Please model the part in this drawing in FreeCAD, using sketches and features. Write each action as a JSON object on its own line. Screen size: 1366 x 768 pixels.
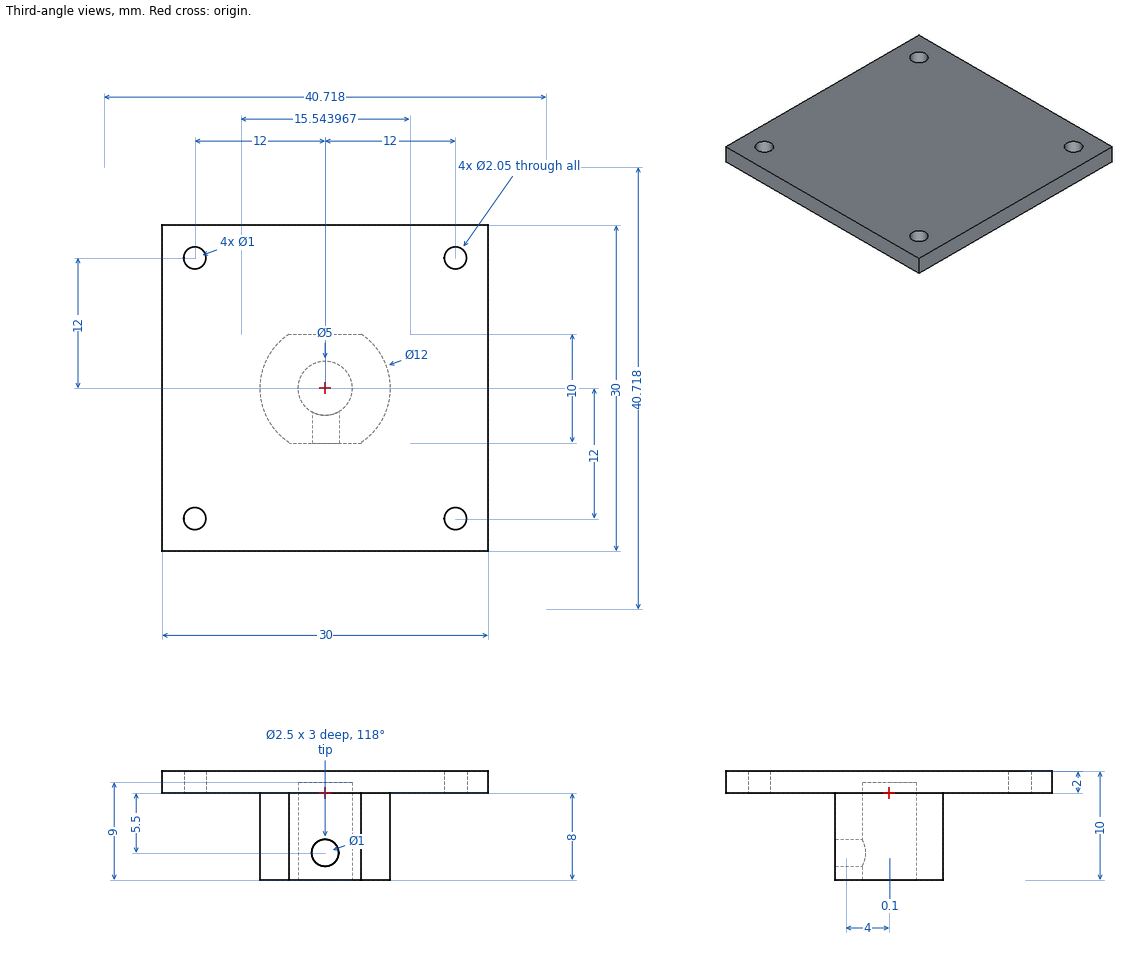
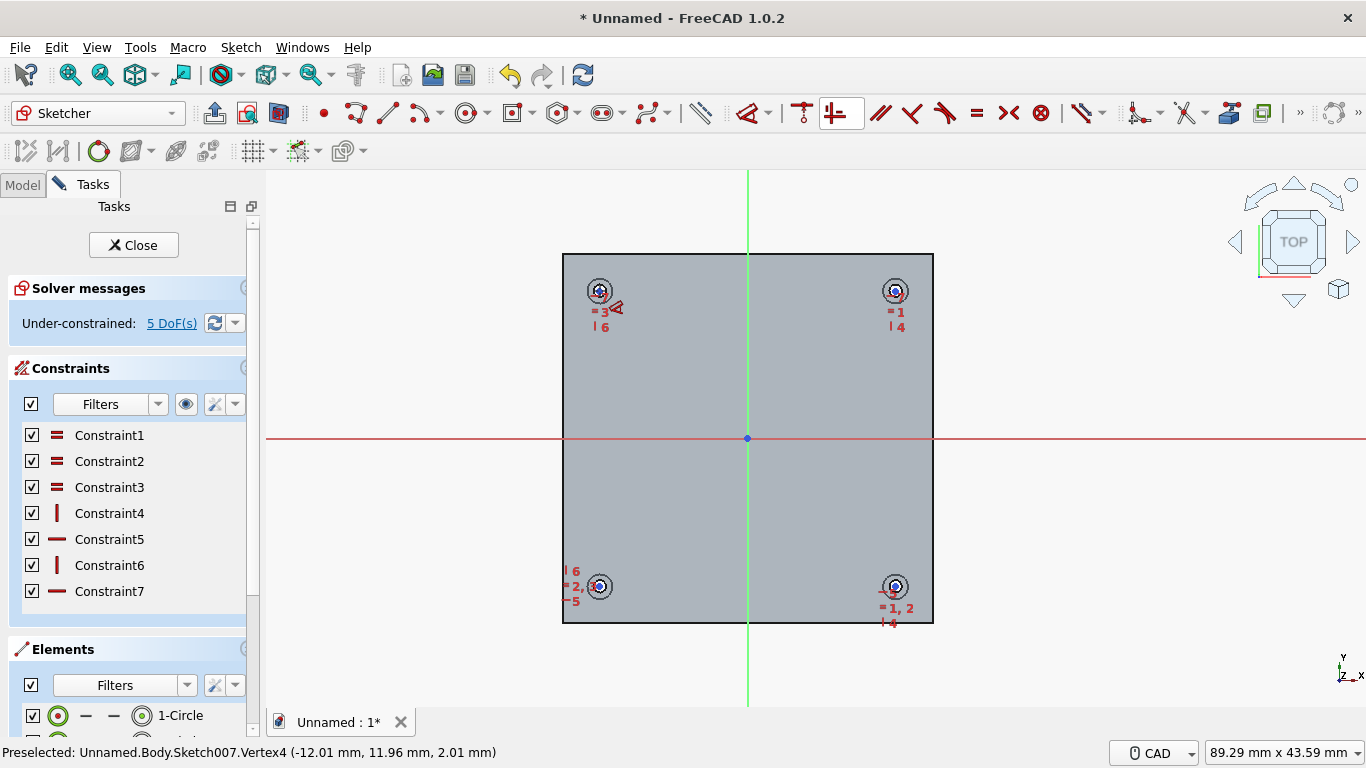
{"action": "scroll", "coordinate": [904, 282], "scroll_direction": "up", "scroll_amount": 3}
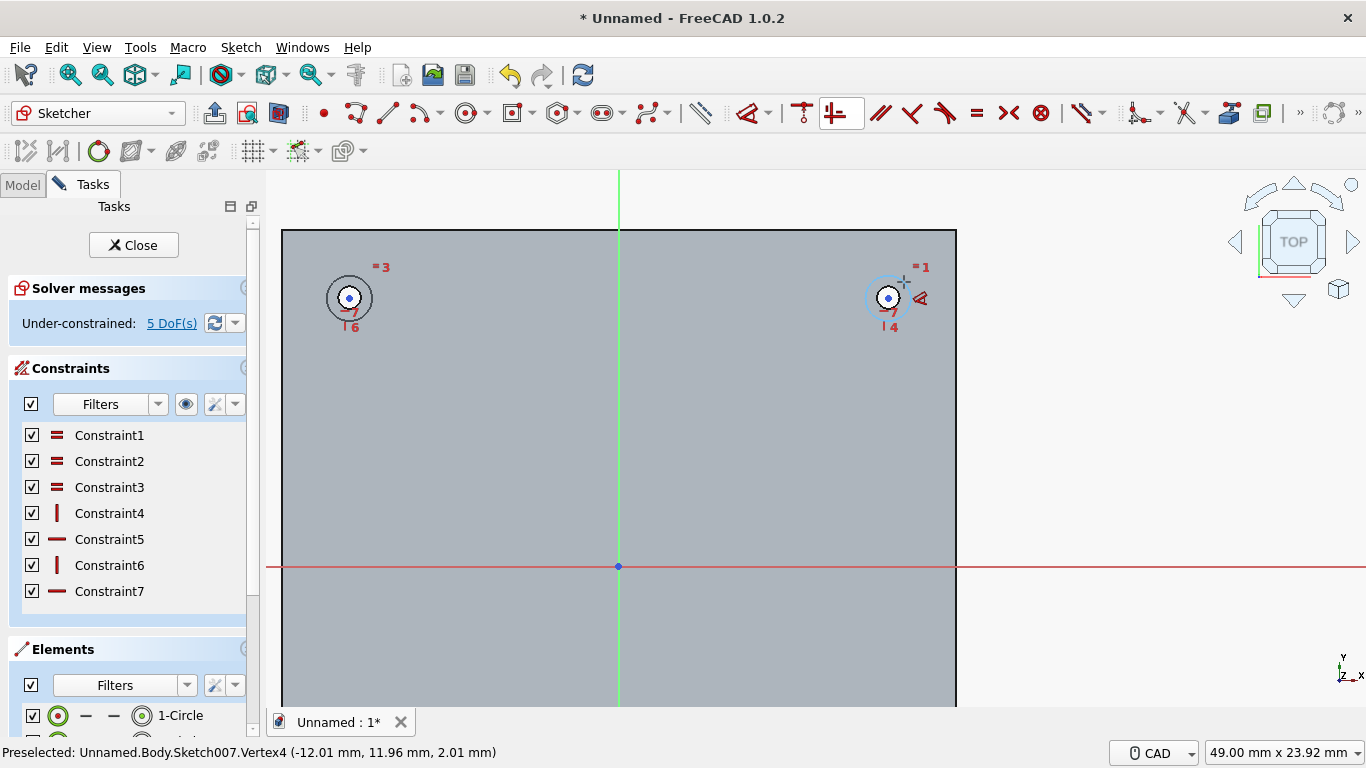
{"action": "left_click", "coordinate": [904, 282]}
{"action": "left_click", "coordinate": [926, 259]}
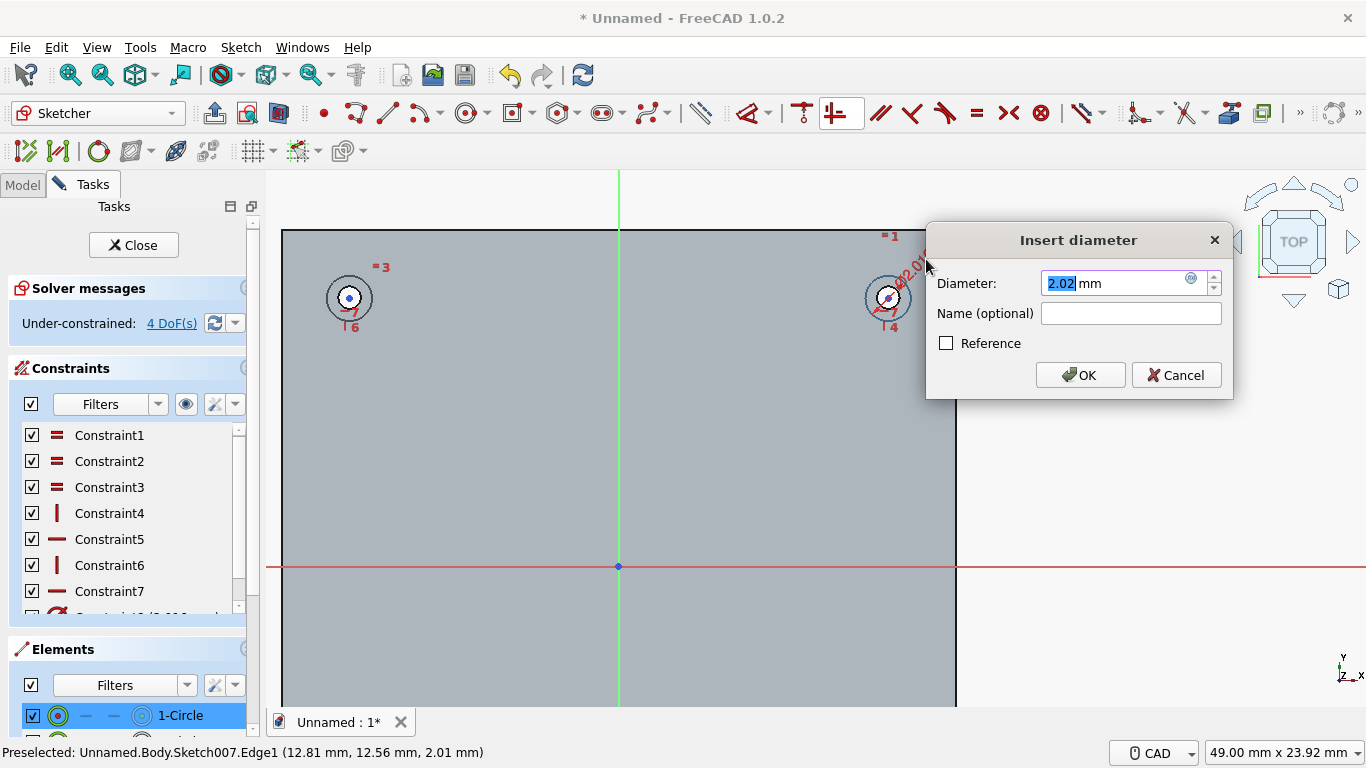
{"action": "type", "text": "2.05"}
{"action": "key", "text": "Return"}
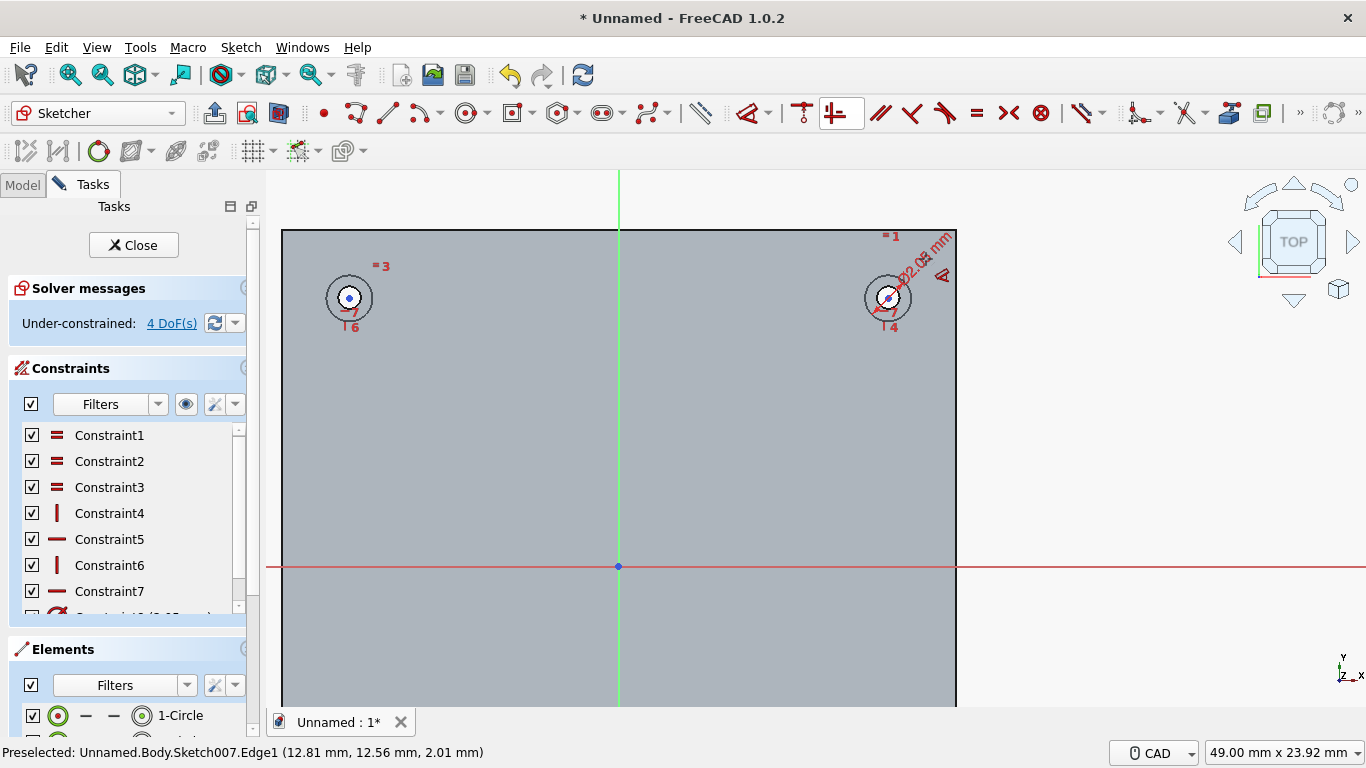
{"action": "left_click", "coordinate": [888, 298]}
{"action": "left_click", "coordinate": [754, 264]}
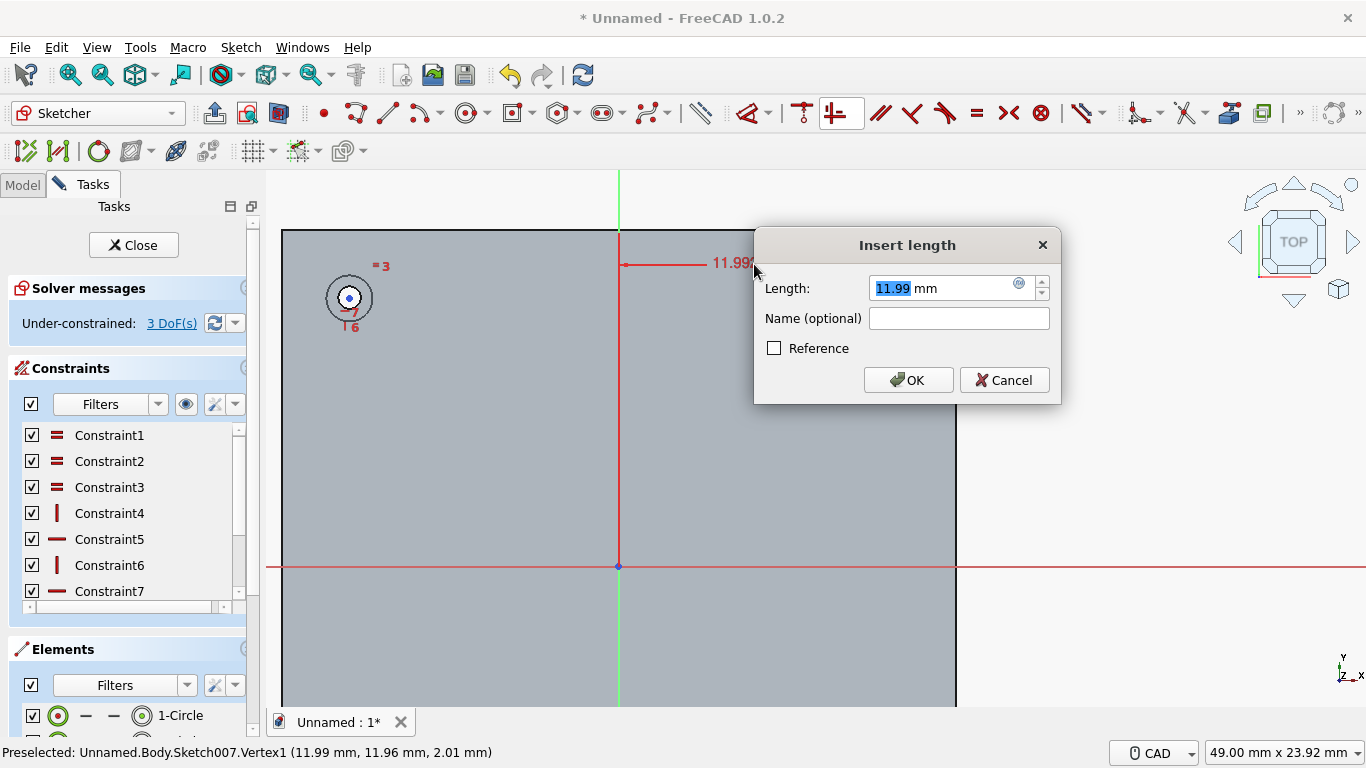
{"action": "type", "text": "12"}
{"action": "key", "text": "Return"}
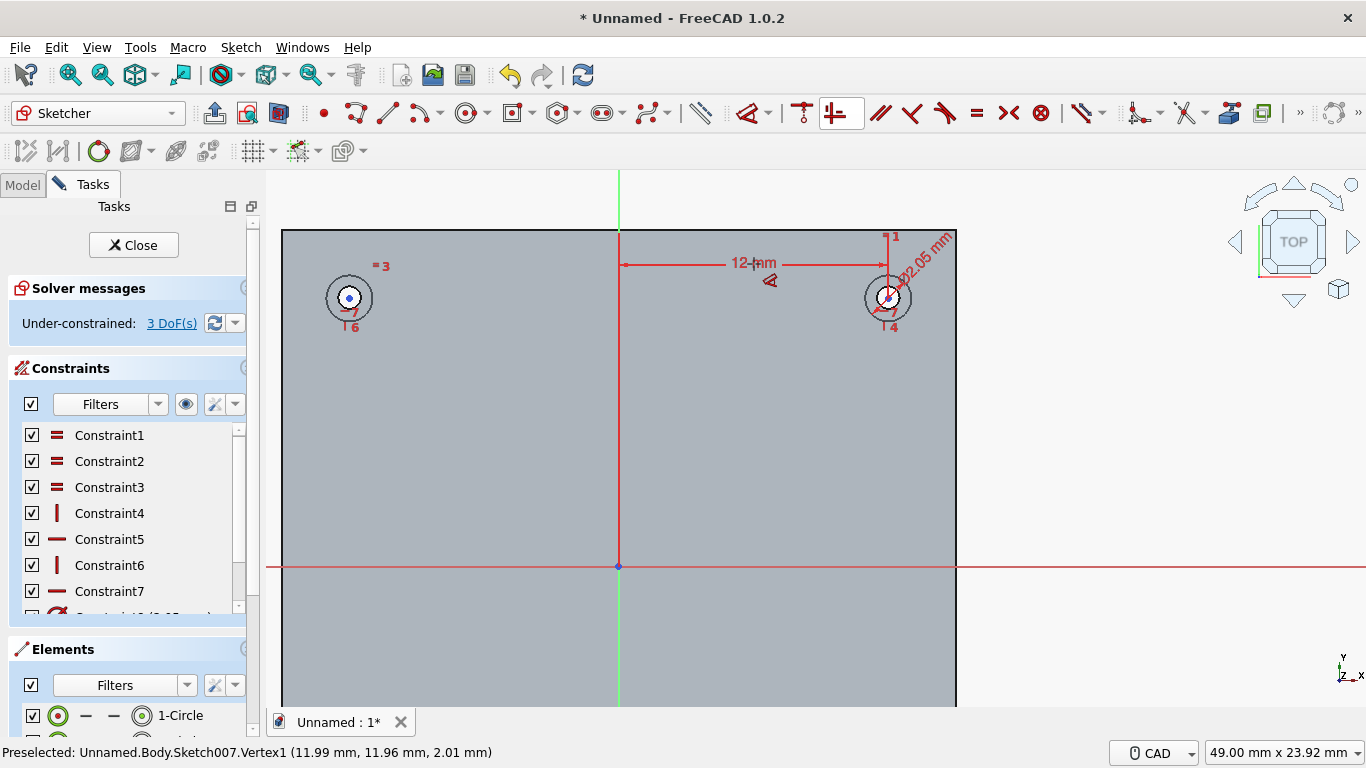
{"action": "left_click", "coordinate": [888, 298]}
{"action": "left_click", "coordinate": [922, 433]}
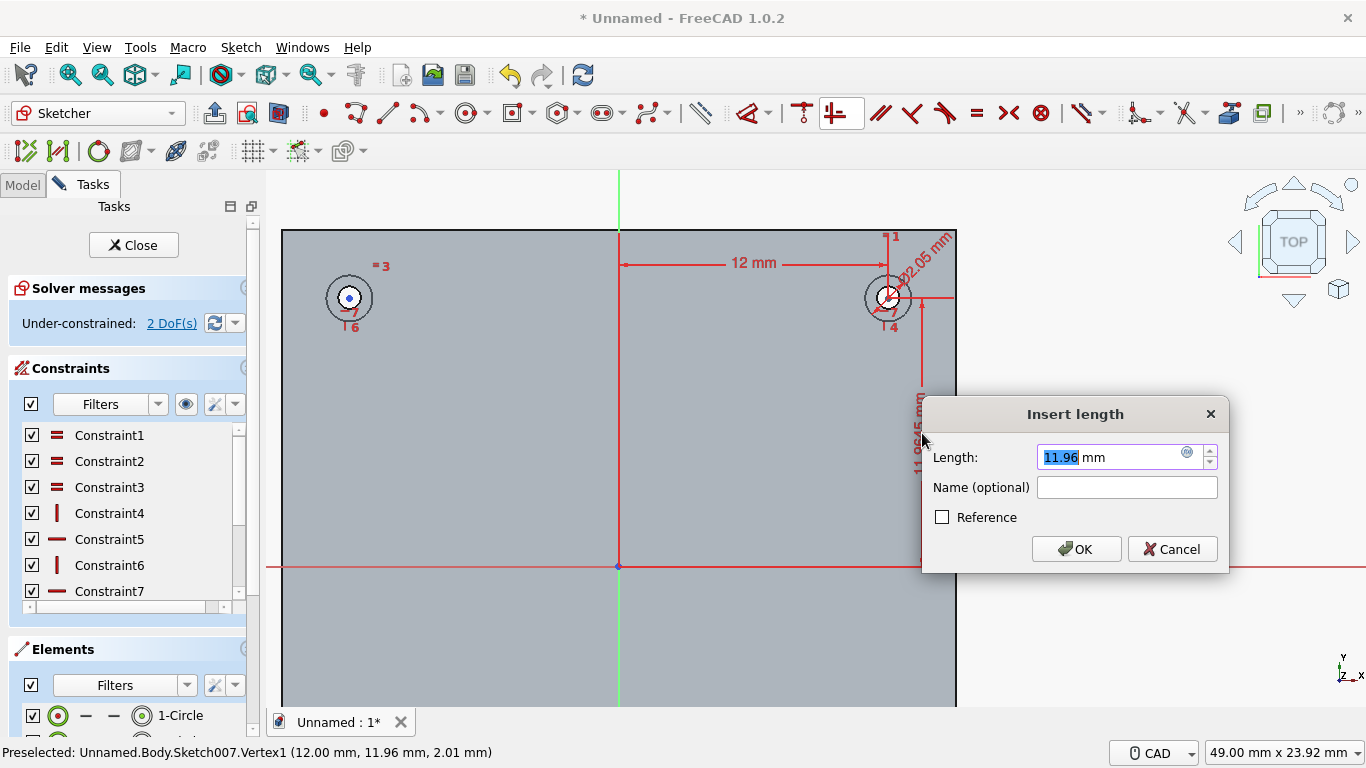
{"action": "type", "text": "12"}
{"action": "key", "text": "Return"}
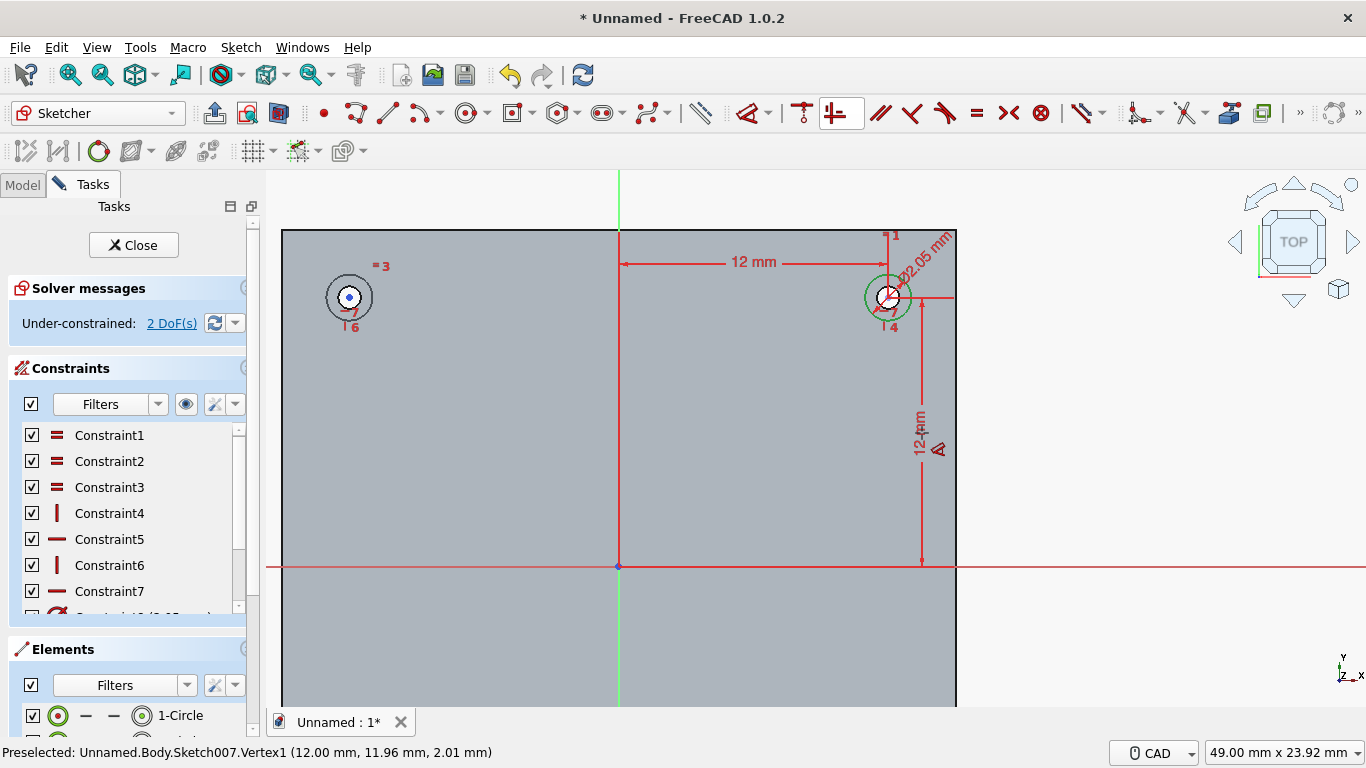
{"action": "scroll", "coordinate": [904, 282], "scroll_direction": "down", "scroll_amount": 3}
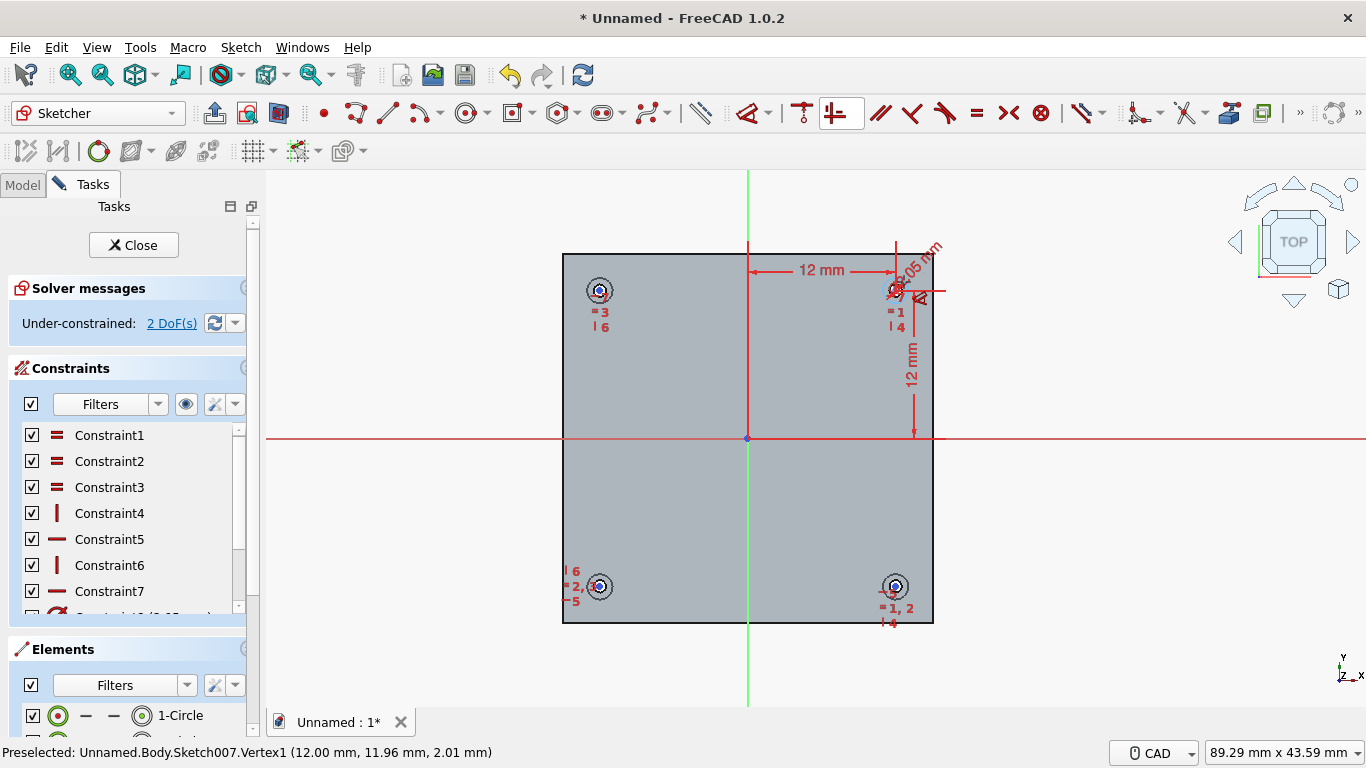
{"action": "left_click", "coordinate": [896, 587]}
{"action": "left_click", "coordinate": [930, 513]}